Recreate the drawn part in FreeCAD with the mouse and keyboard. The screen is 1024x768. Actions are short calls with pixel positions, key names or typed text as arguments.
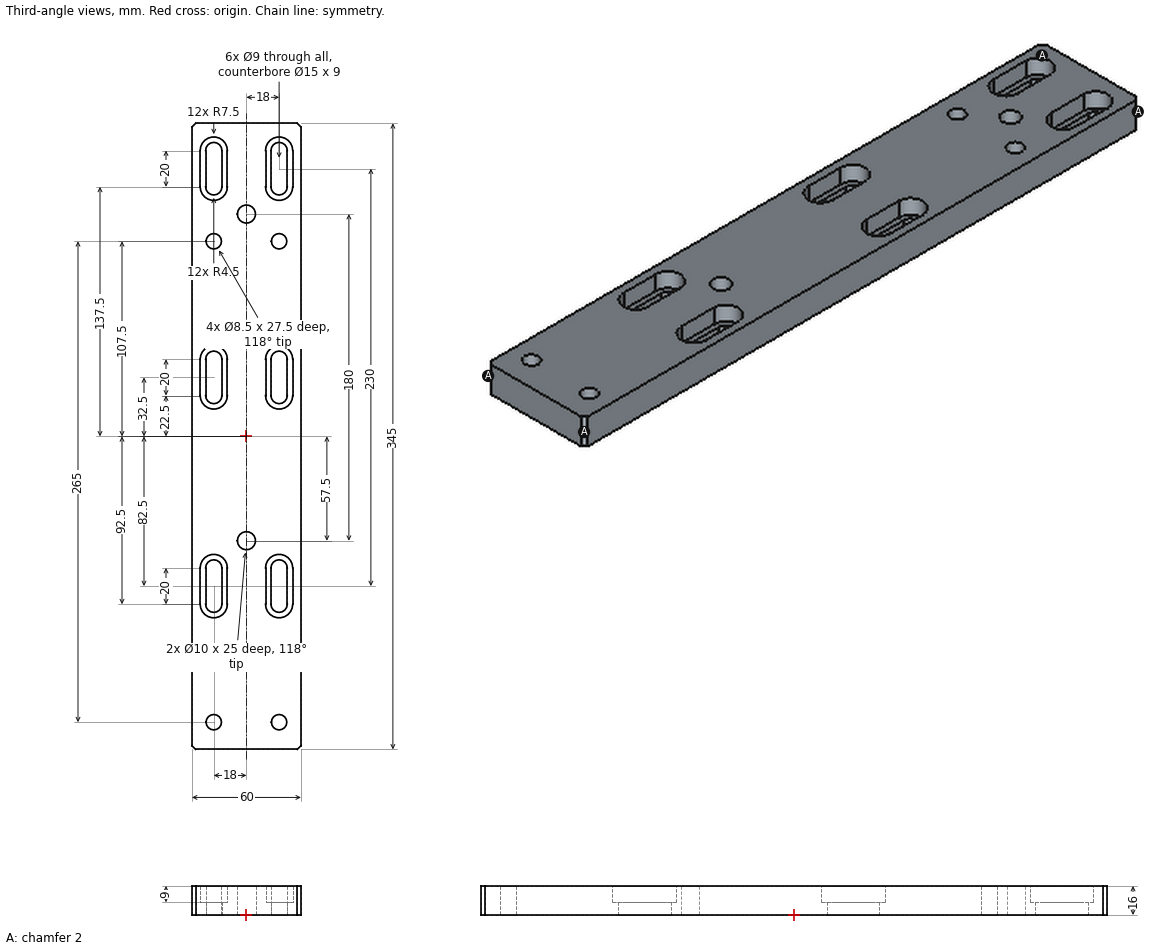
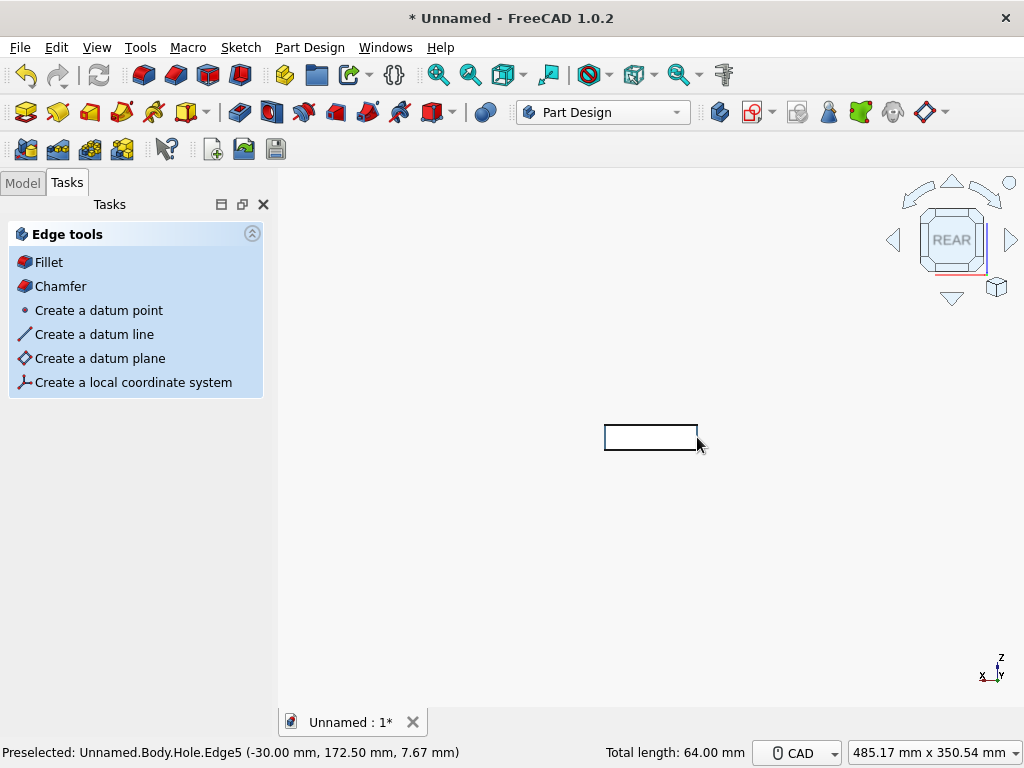
click(176, 76)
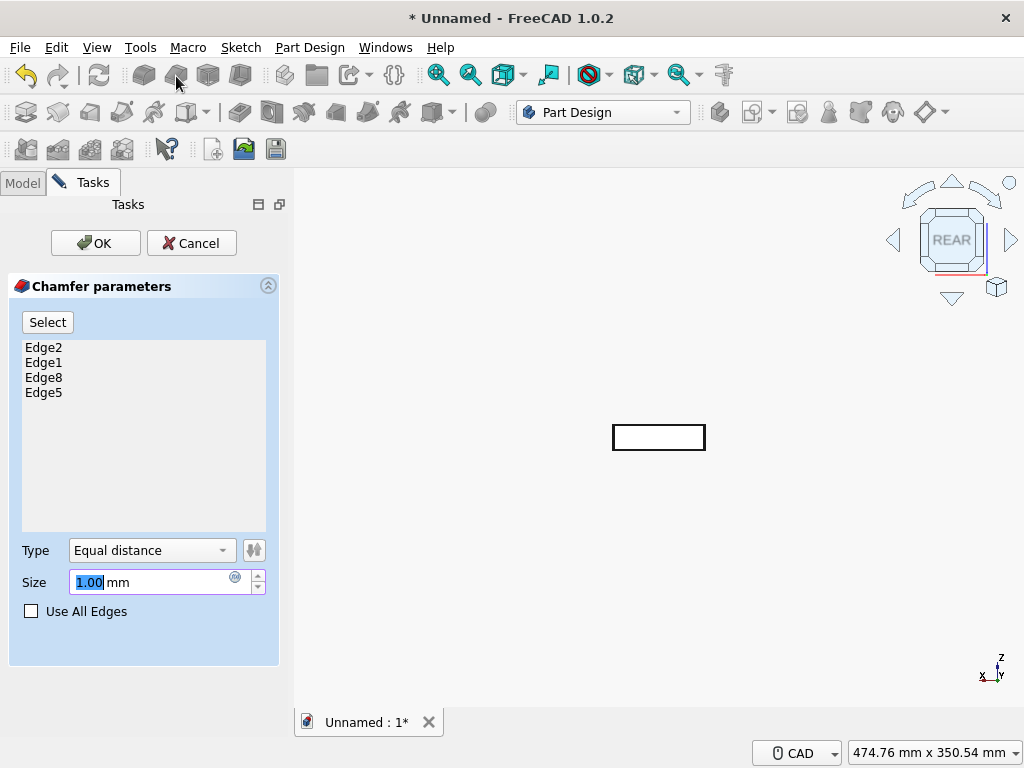
text(2)
key(Tab)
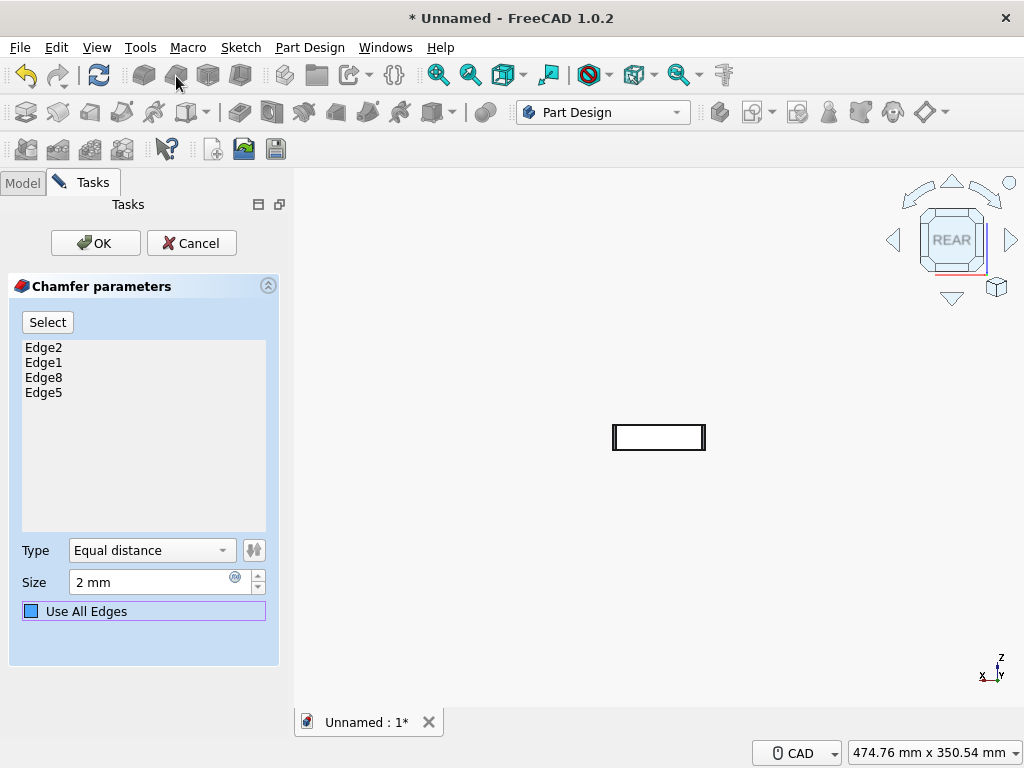
click(96, 243)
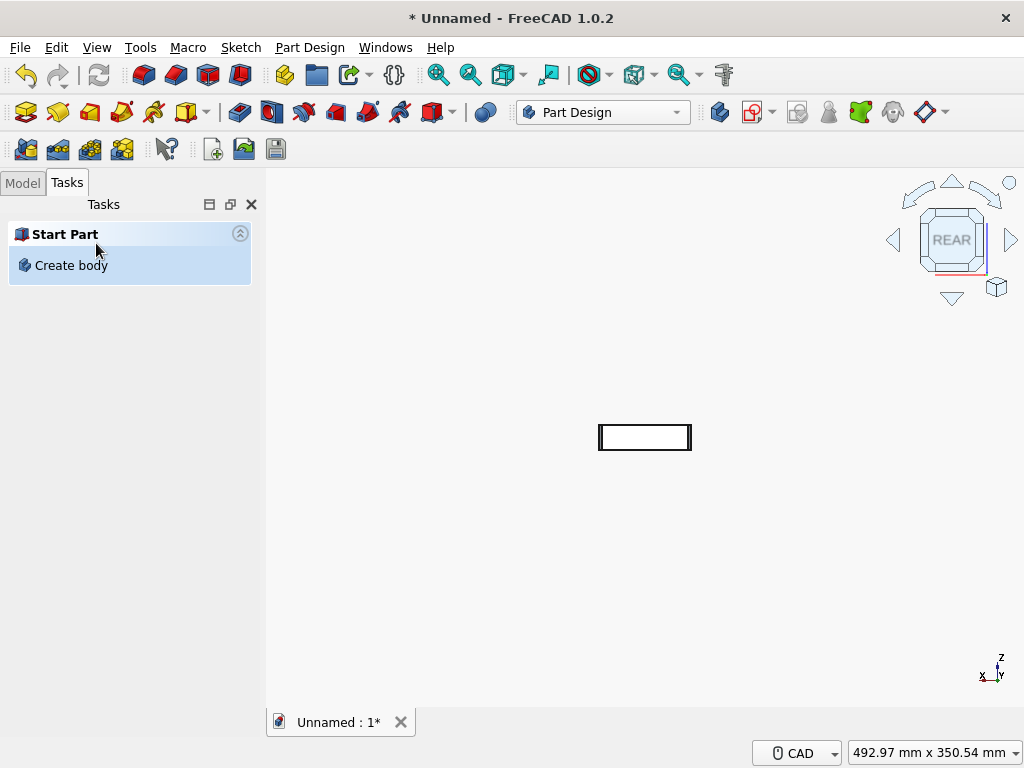
key(v)
key(f)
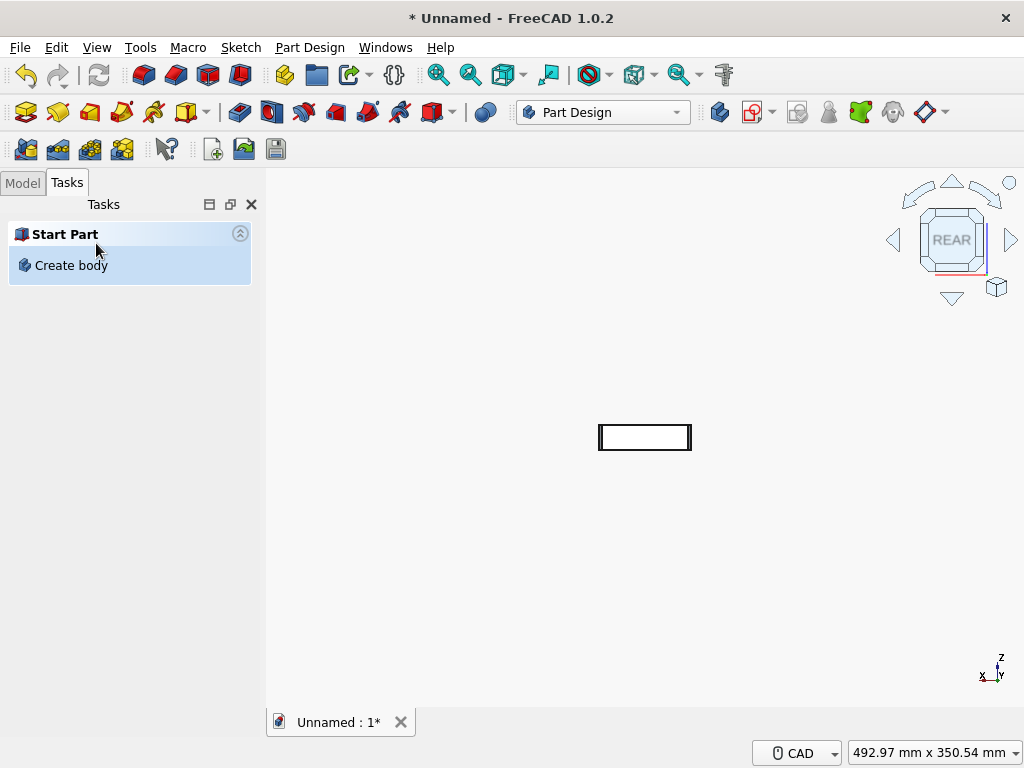
key(0)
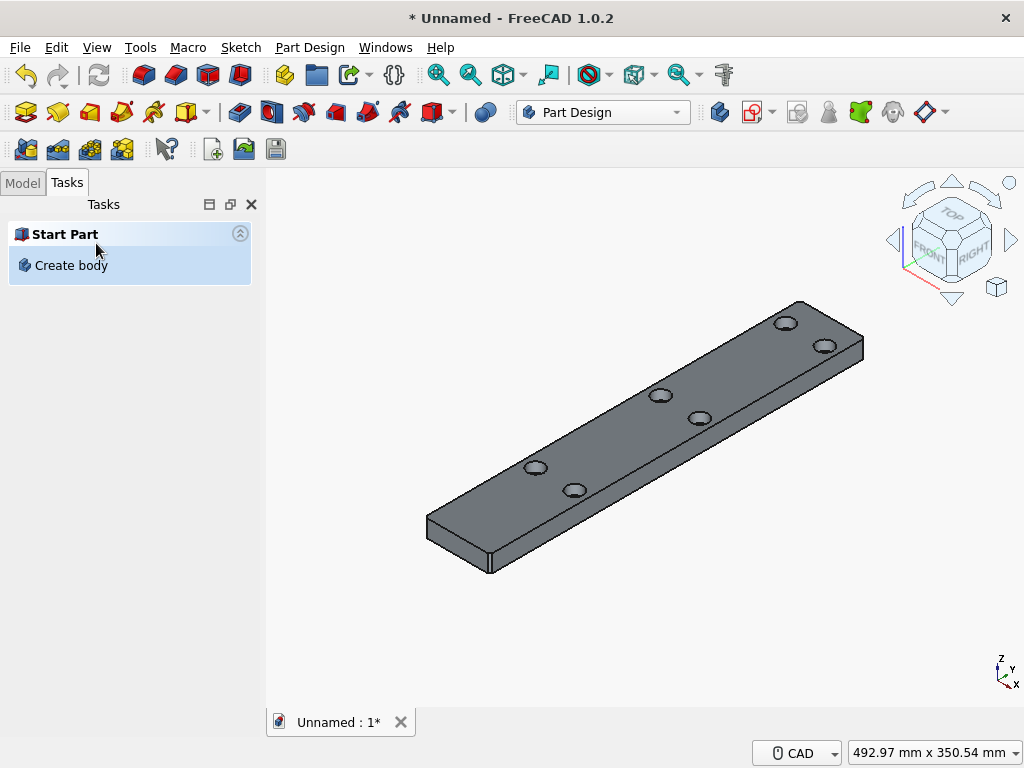
click(752, 365)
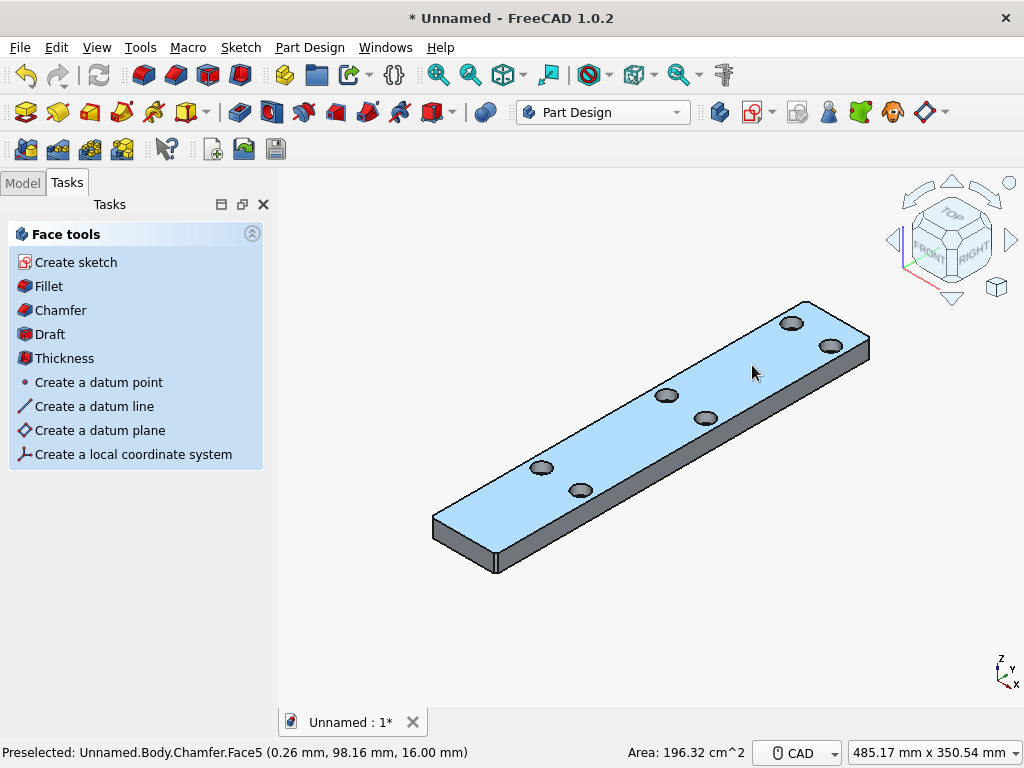
click(752, 112)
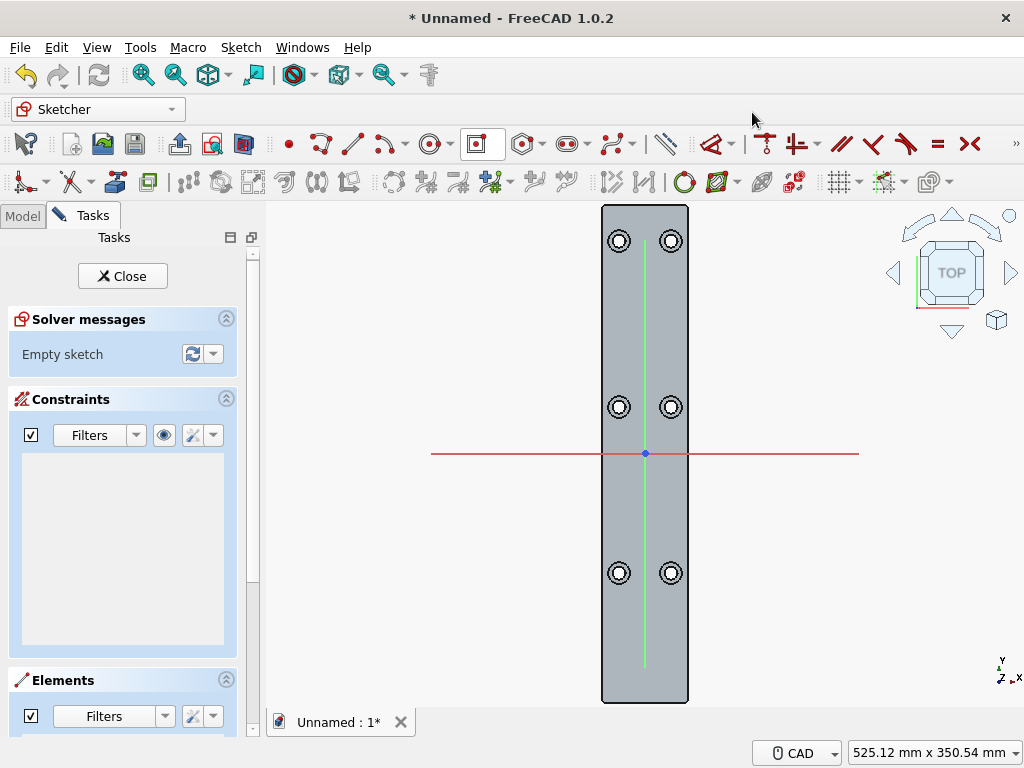
scroll(294, 666, down, 1)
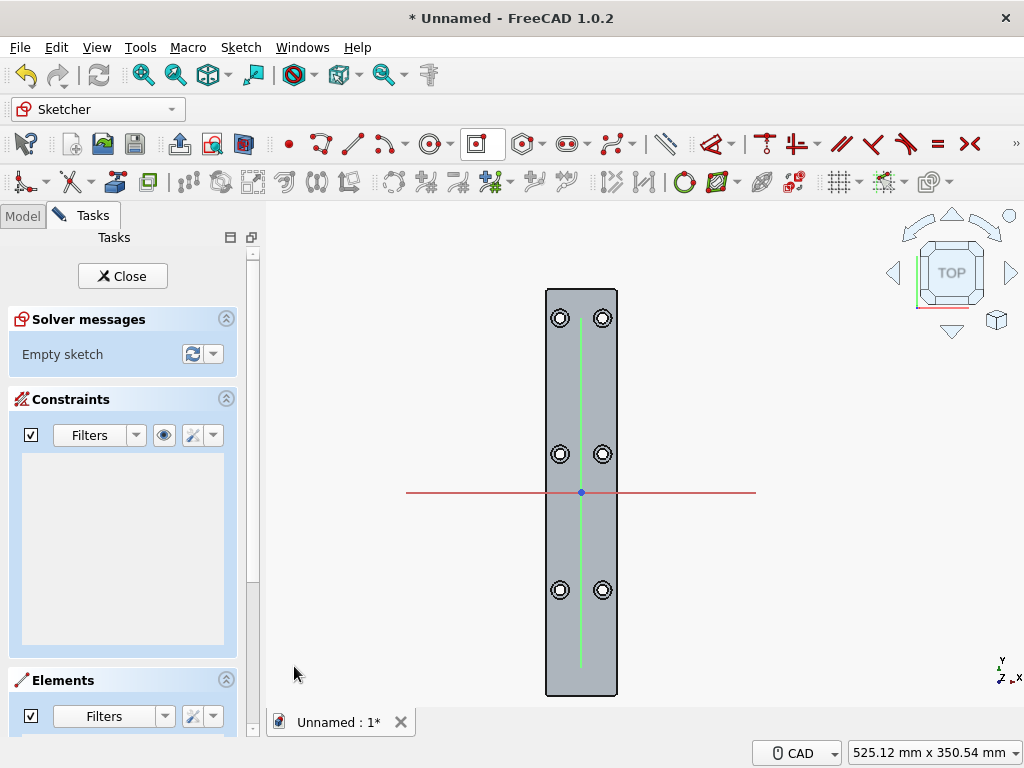
key(g)
key(s)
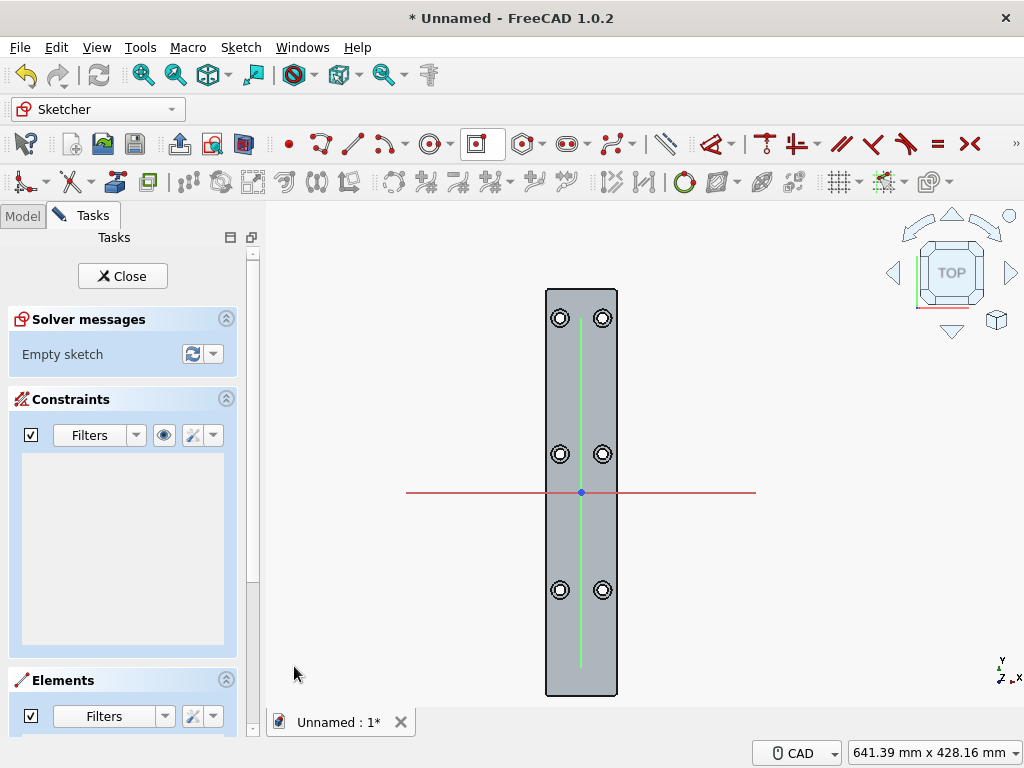
scroll(560, 330, up, 5)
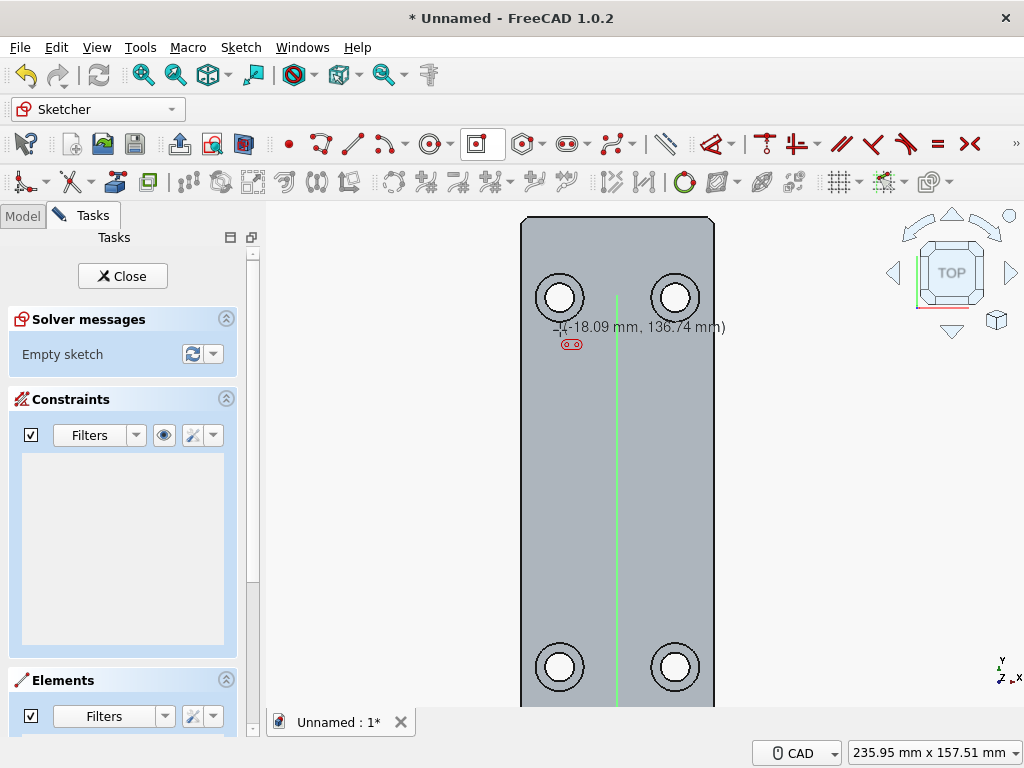
click(560, 330)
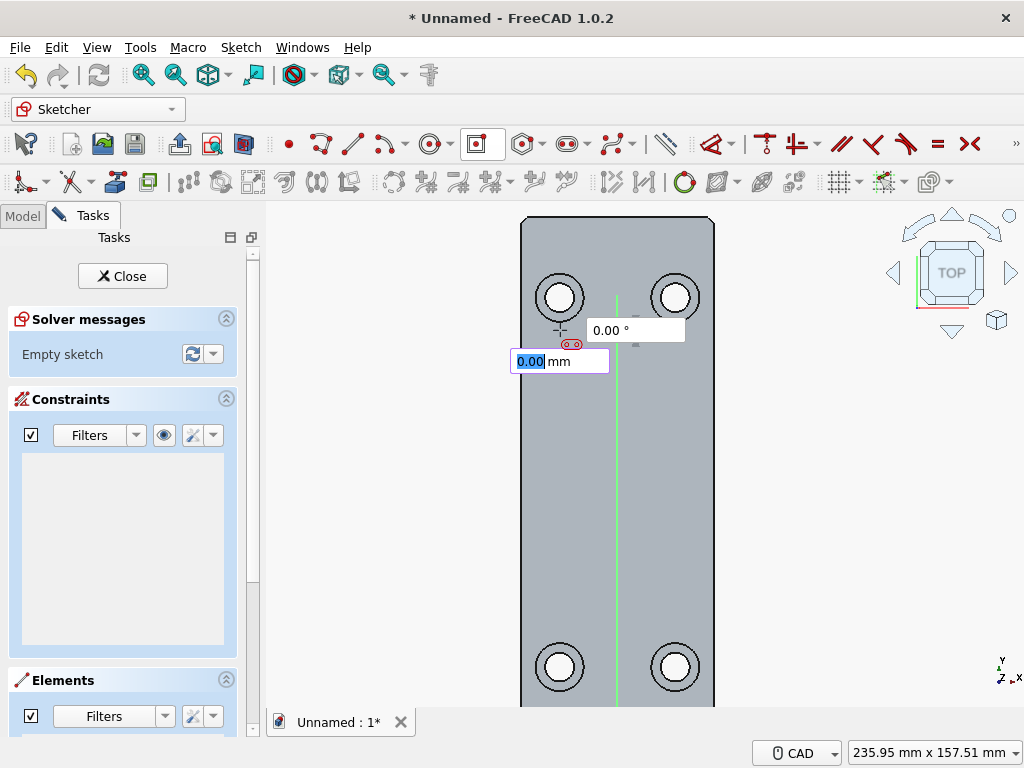
click(560, 266)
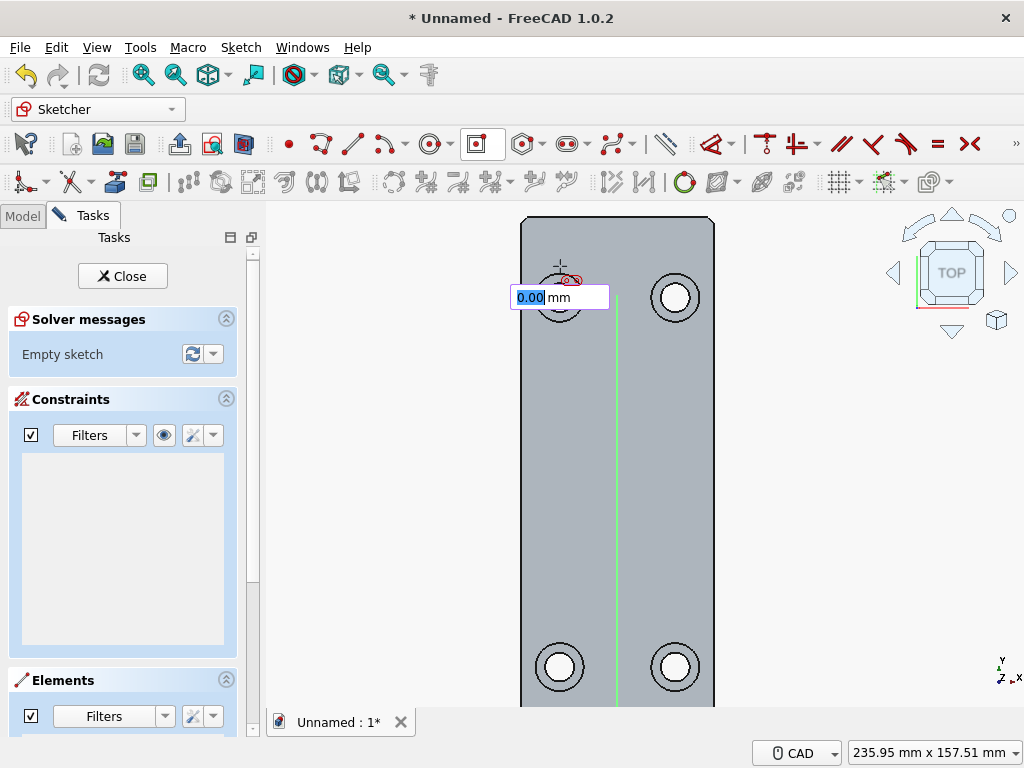
click(584, 298)